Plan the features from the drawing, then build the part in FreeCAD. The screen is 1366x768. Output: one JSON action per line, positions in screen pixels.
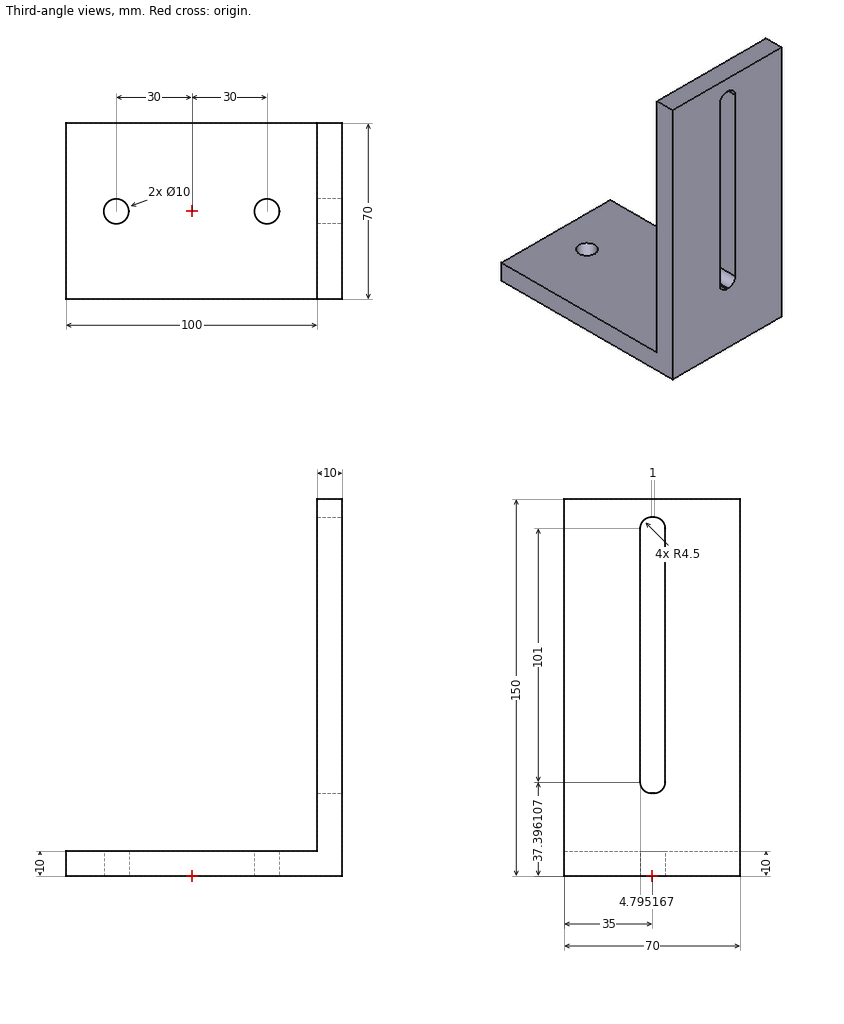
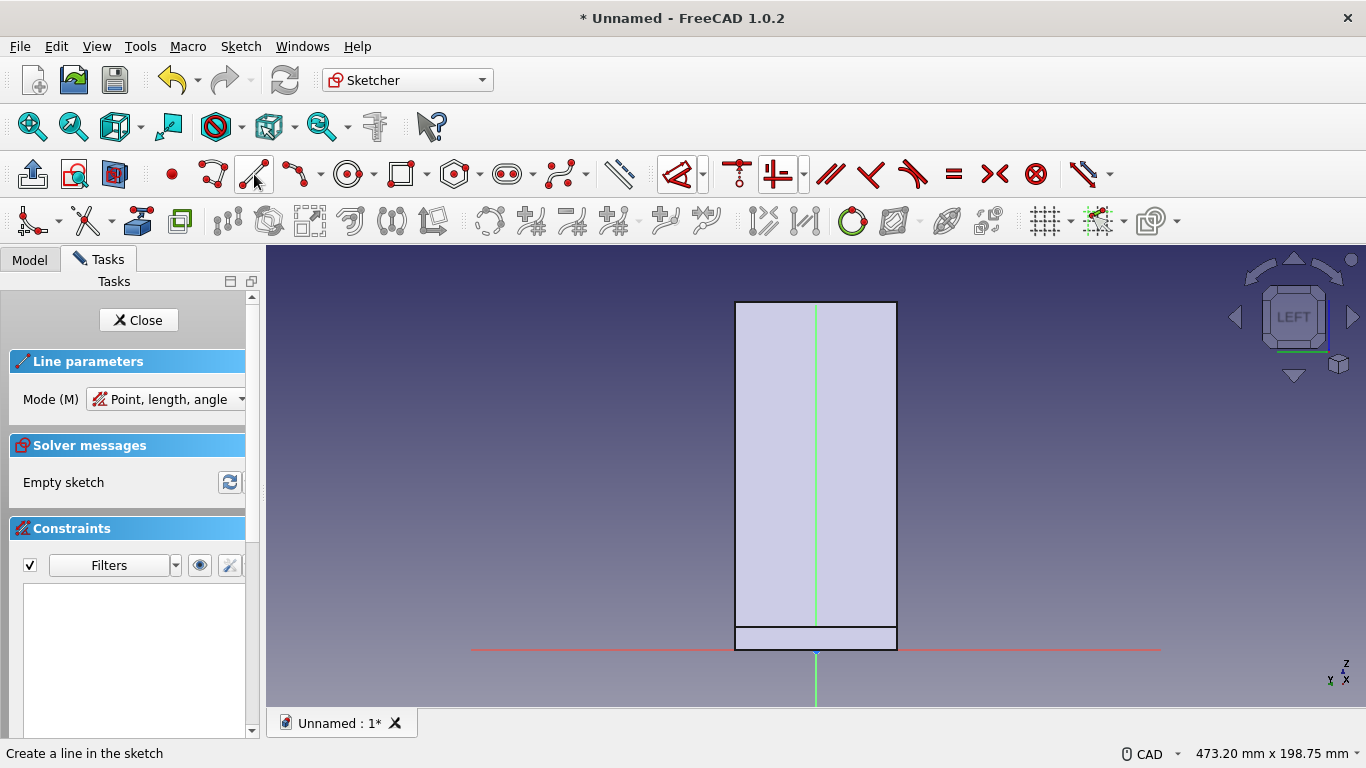
{"action": "scroll", "coordinate": [827, 563], "scroll_direction": "up", "scroll_amount": 2}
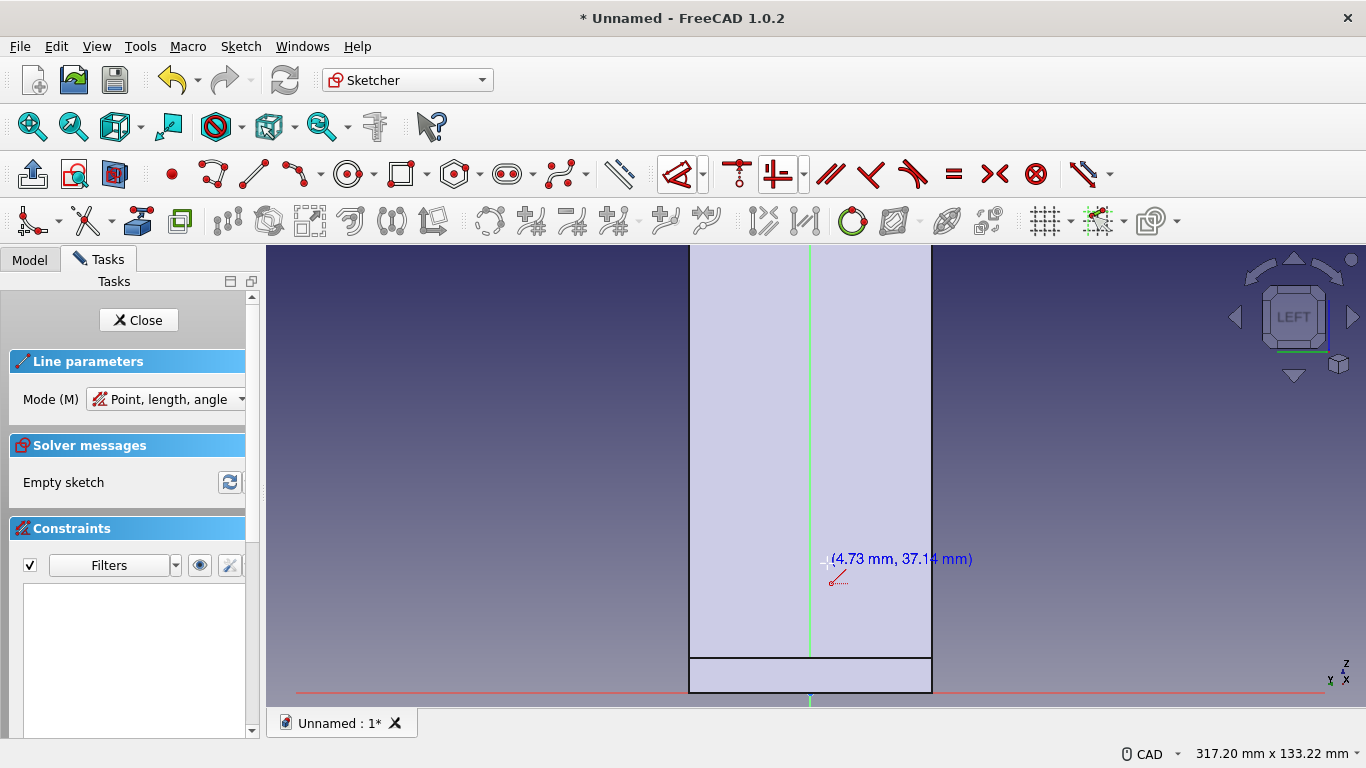
{"action": "left_click", "coordinate": [827, 563]}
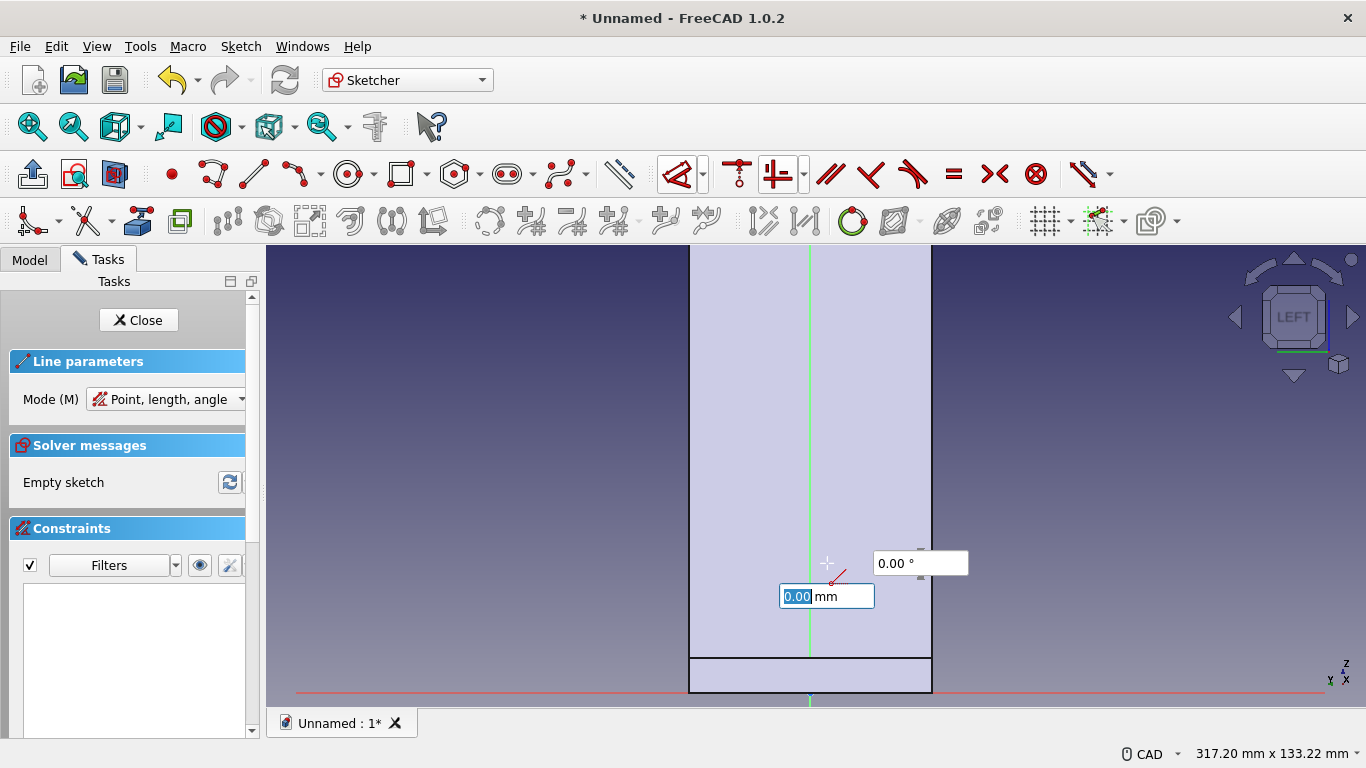
{"action": "scroll", "coordinate": [672, 513], "scroll_direction": "down", "scroll_amount": 3}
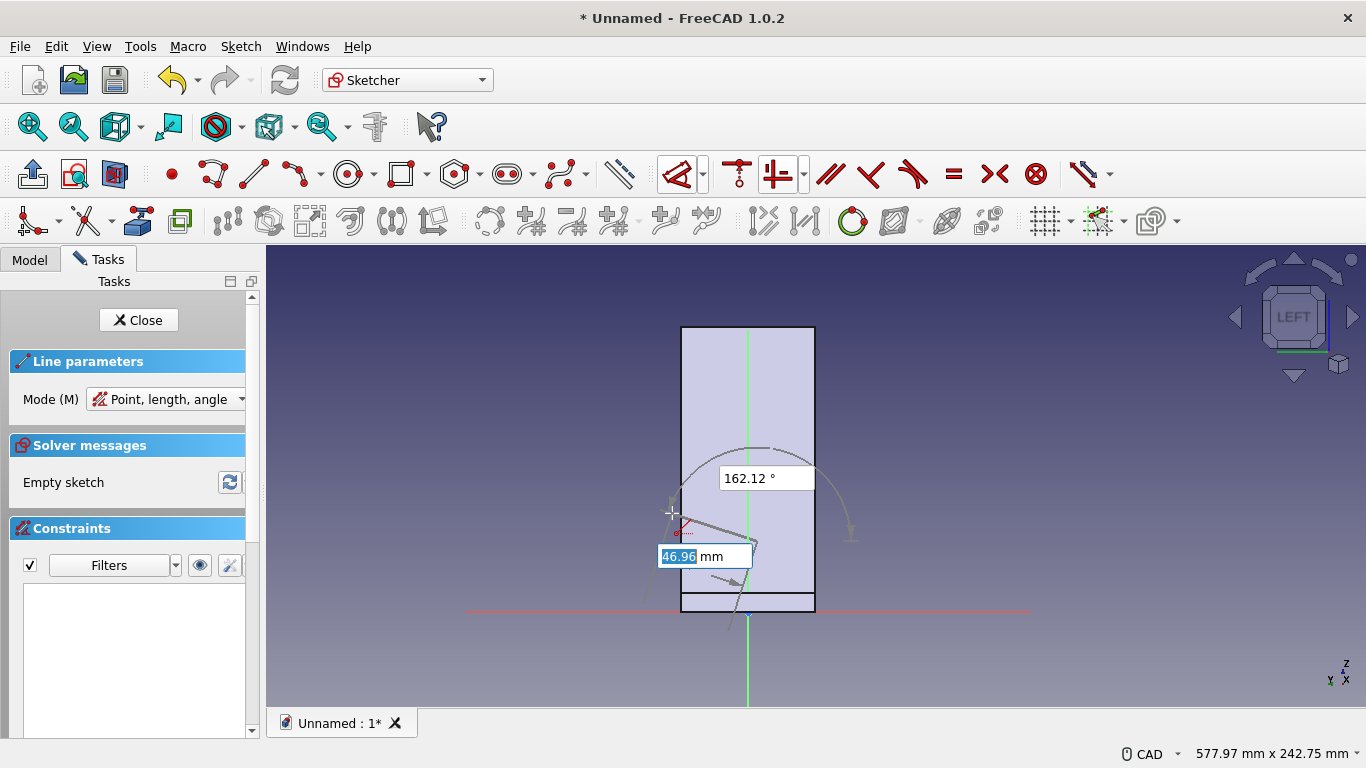
{"action": "scroll", "coordinate": [757, 349], "scroll_direction": "up", "scroll_amount": 3}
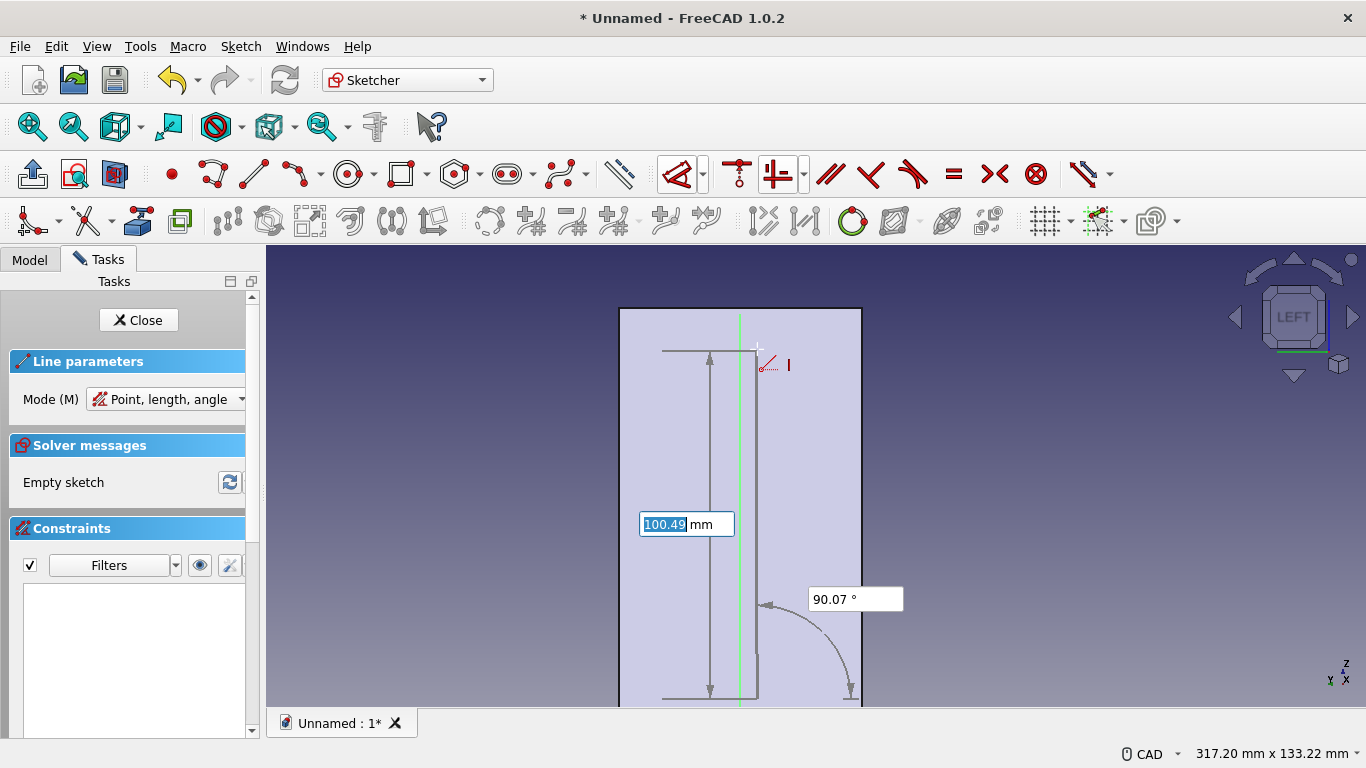
{"action": "left_click", "coordinate": [757, 348]}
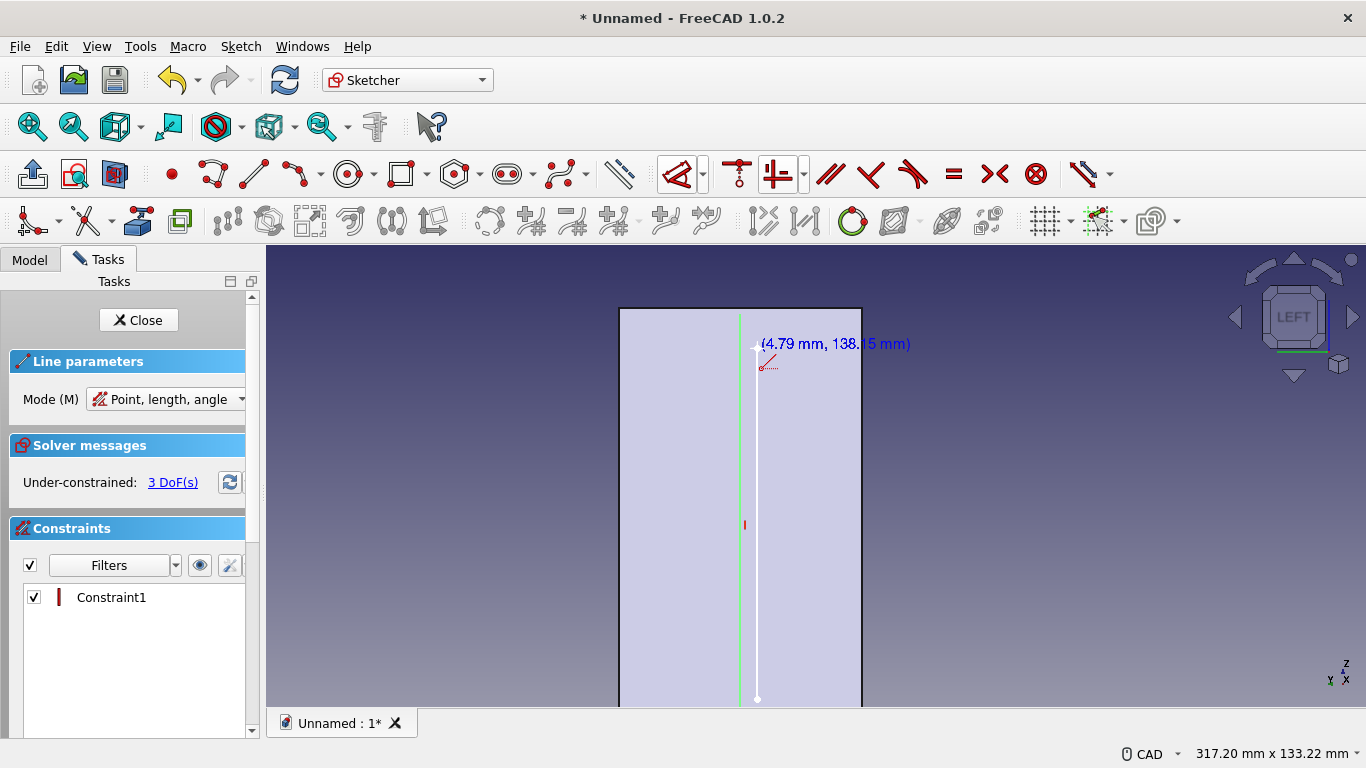
{"action": "scroll", "coordinate": [741, 333], "scroll_direction": "up", "scroll_amount": 14}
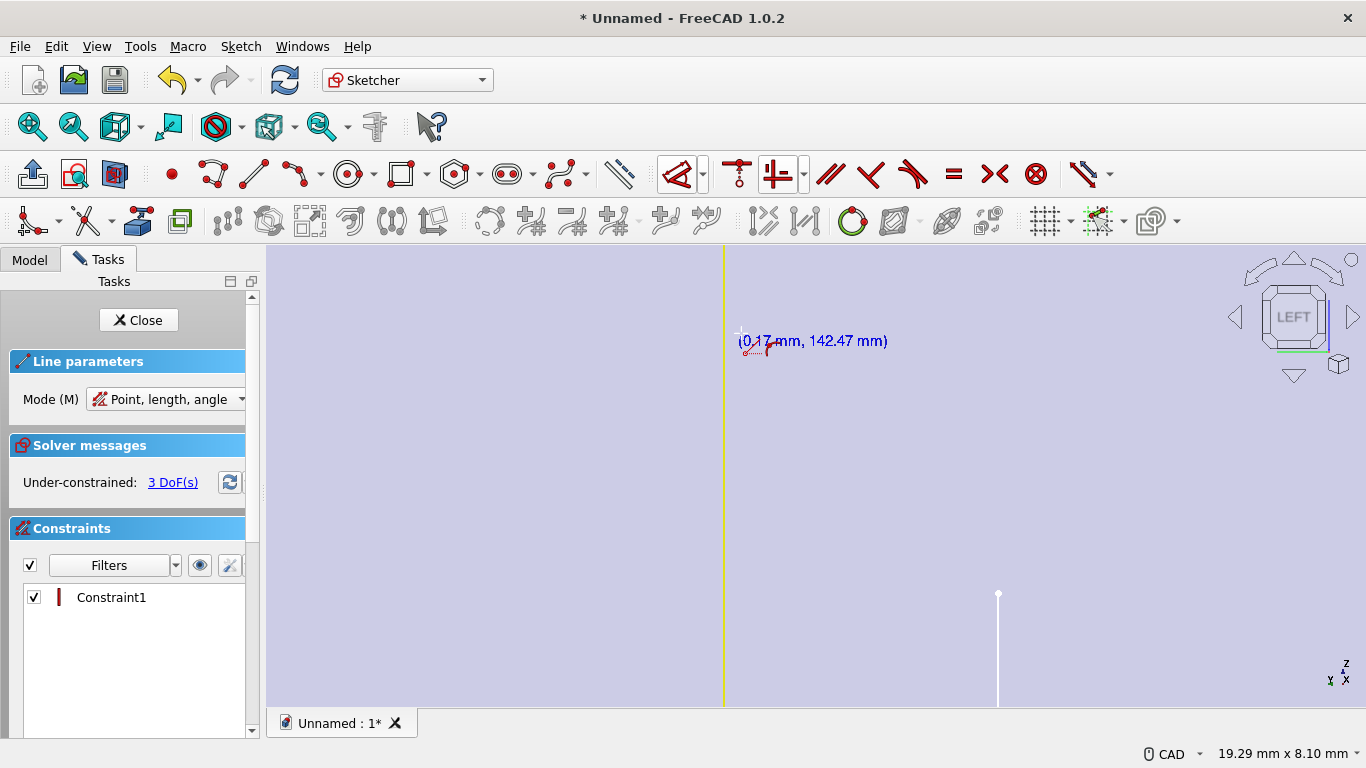
{"action": "left_click", "coordinate": [741, 322]}
{"action": "left_click", "coordinate": [684, 322]}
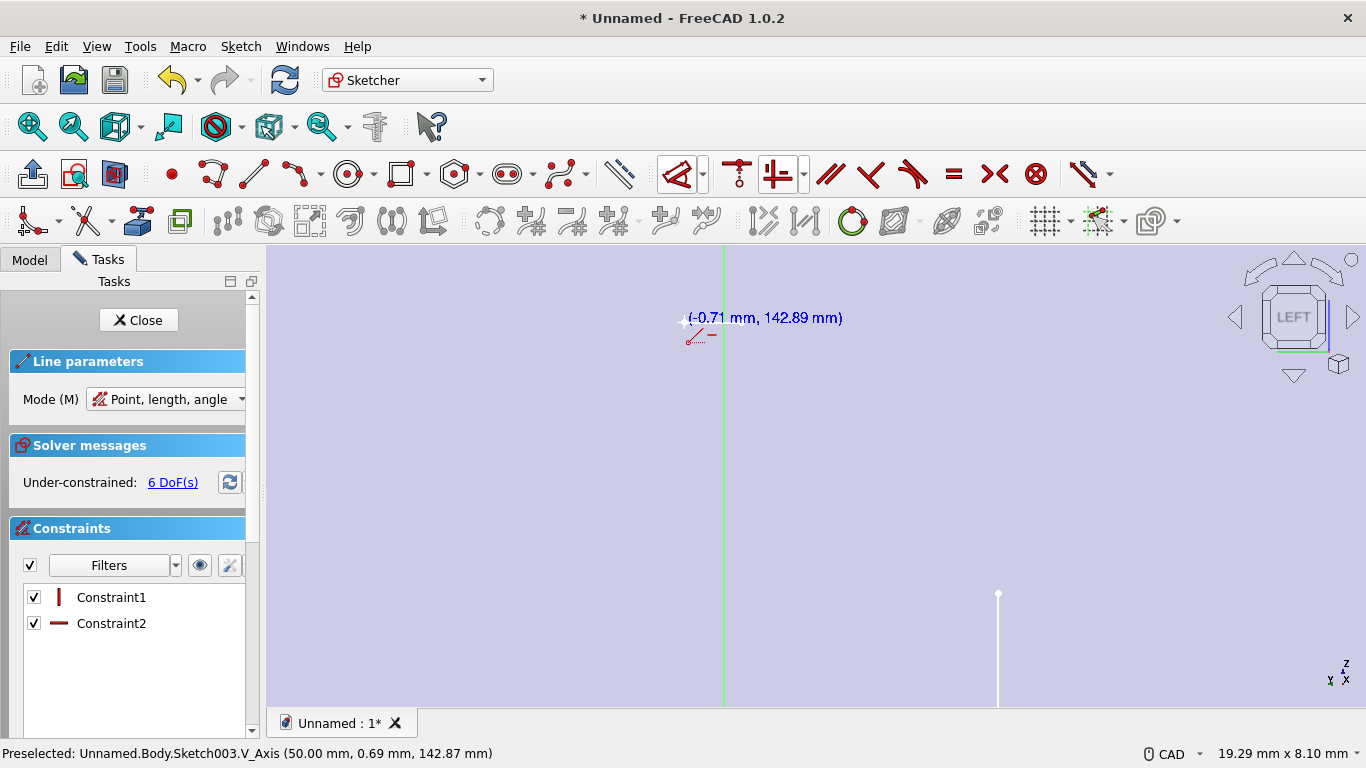
{"action": "scroll", "coordinate": [749, 309], "scroll_direction": "down", "scroll_amount": 16}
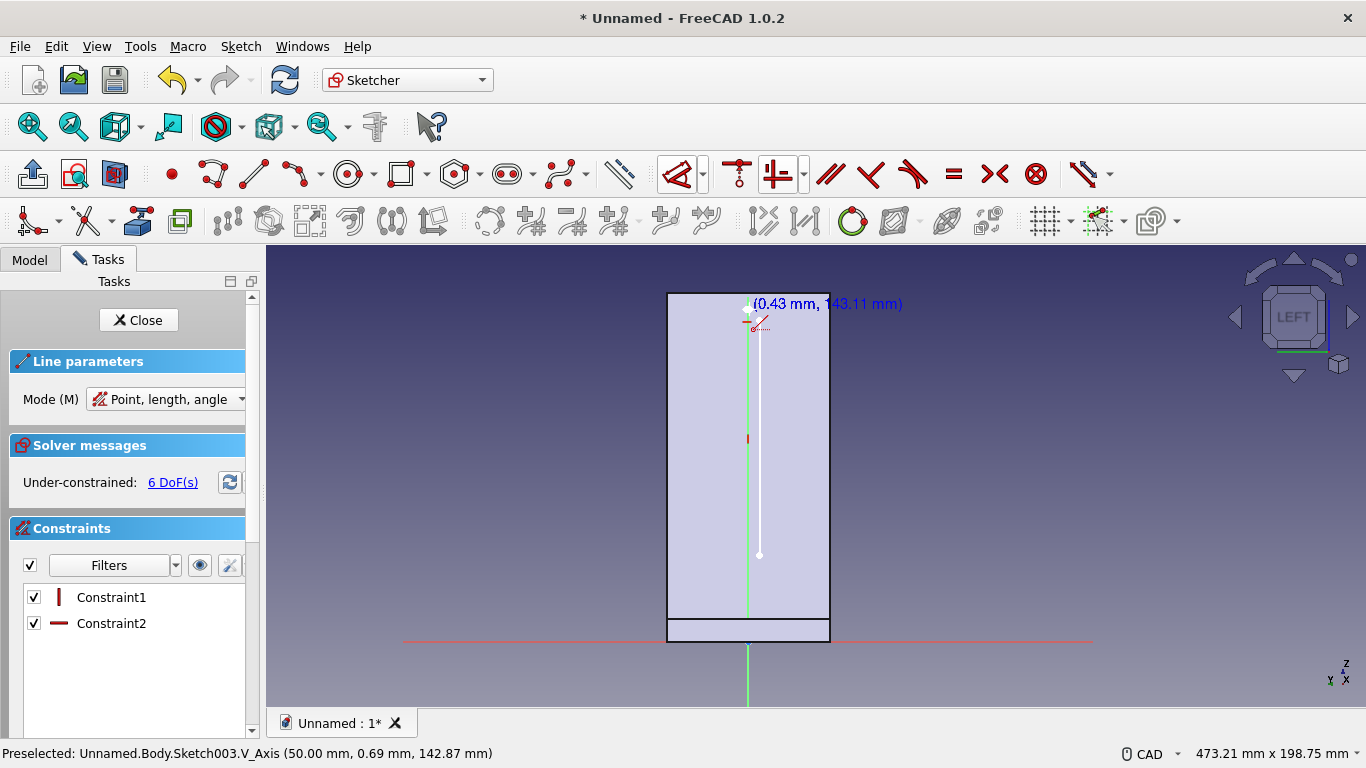
{"action": "scroll", "coordinate": [736, 320], "scroll_direction": "up", "scroll_amount": 2}